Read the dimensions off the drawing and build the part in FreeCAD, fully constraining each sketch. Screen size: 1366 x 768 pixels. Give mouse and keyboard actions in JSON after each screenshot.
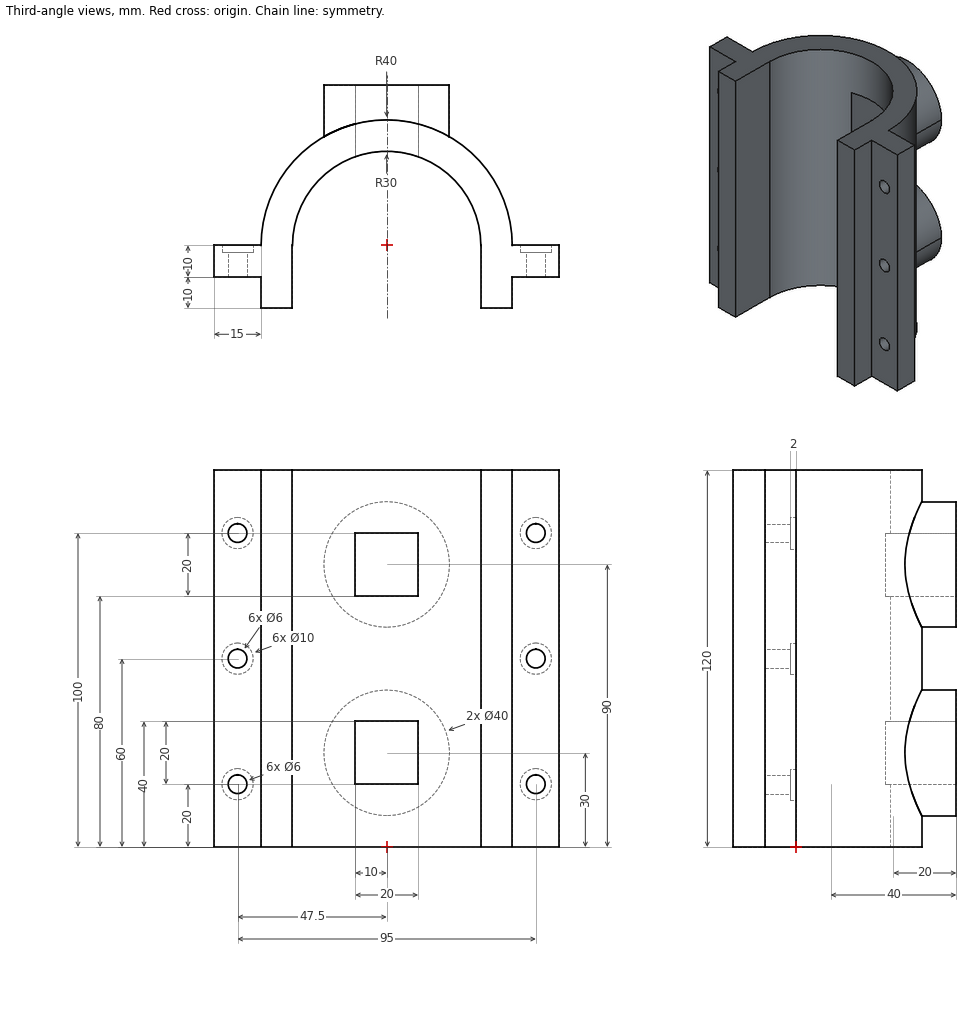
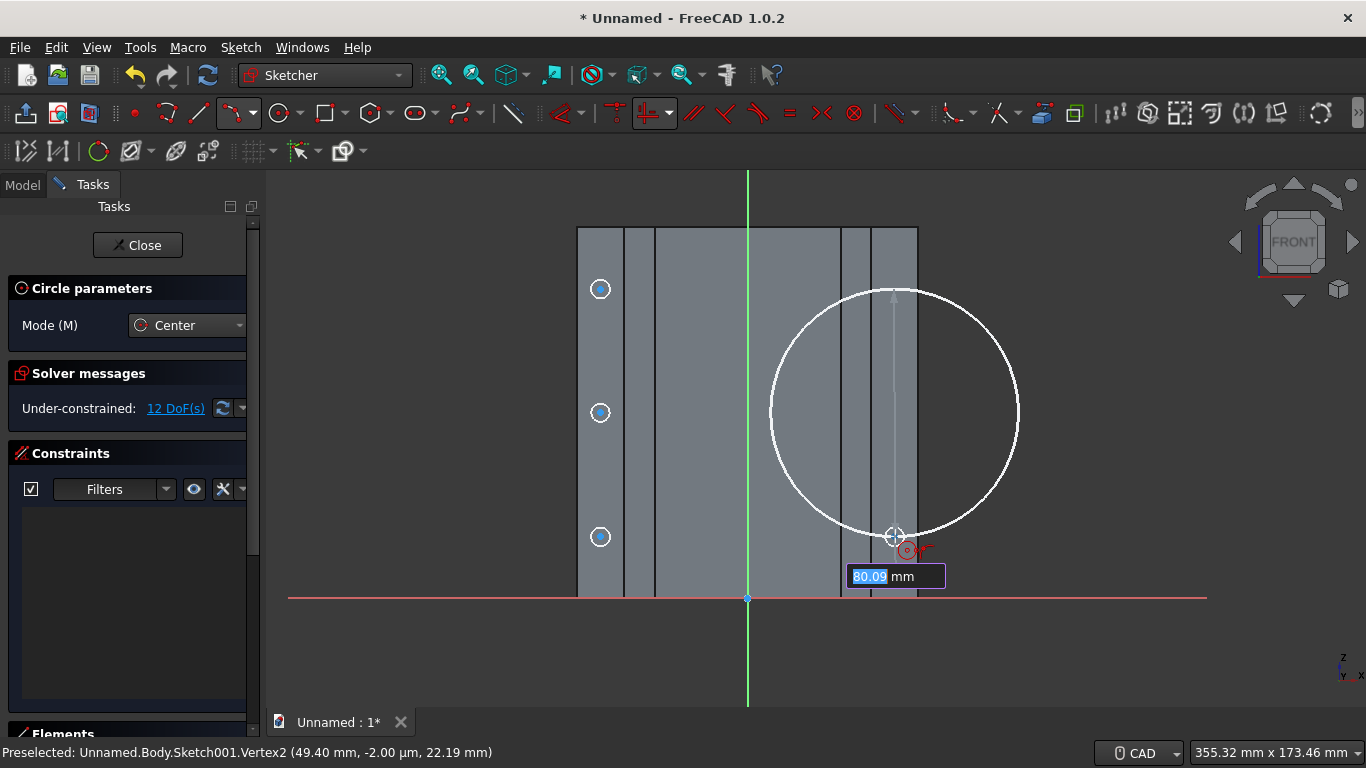
{"action": "scroll", "coordinate": [901, 406], "scroll_direction": "up", "scroll_amount": 3}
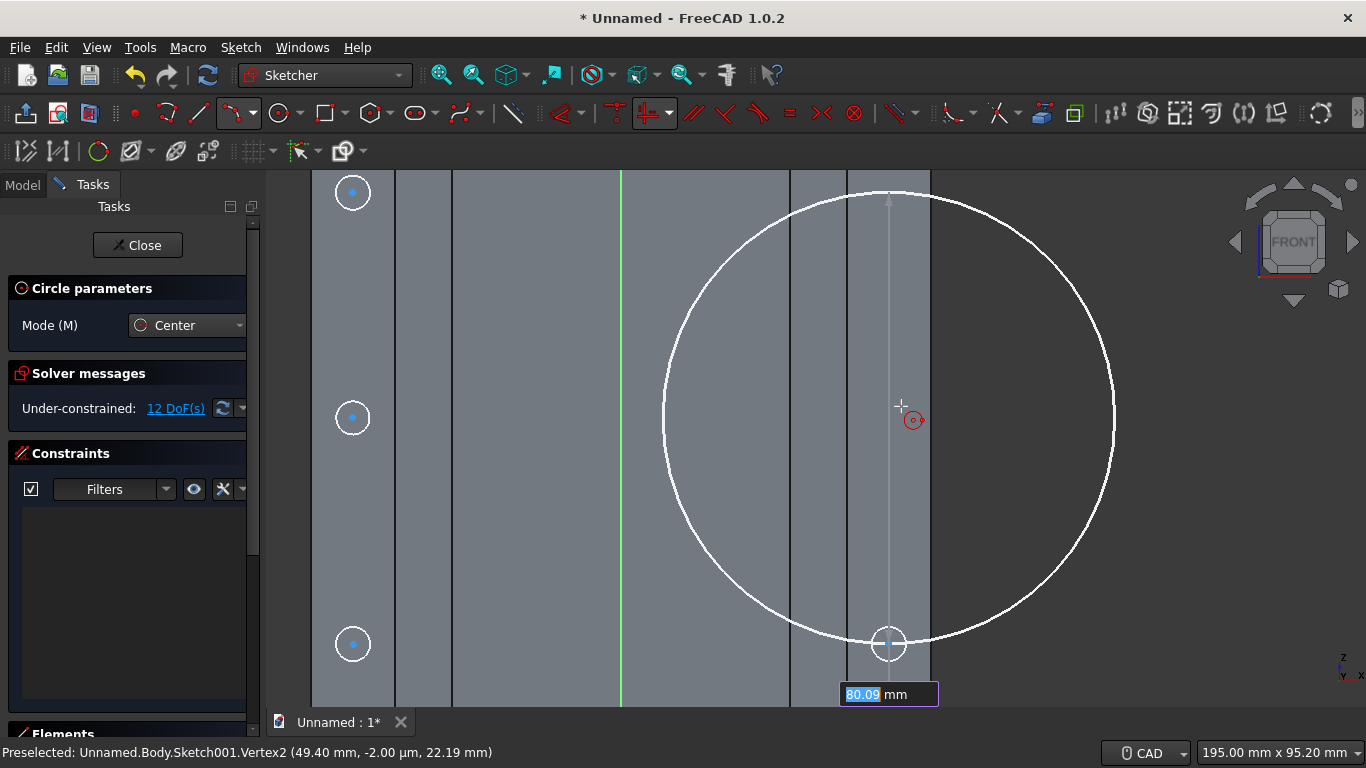
{"action": "left_click", "coordinate": [901, 406]}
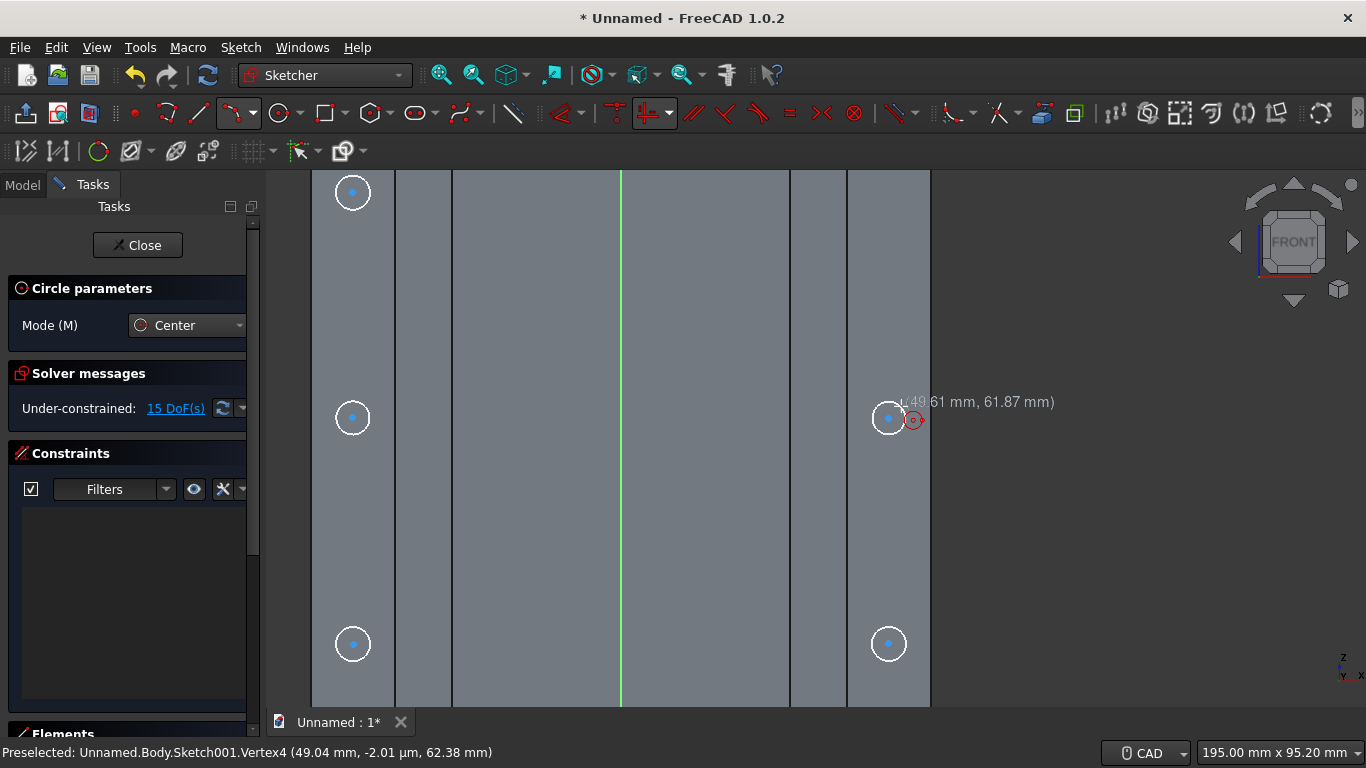
{"action": "scroll", "coordinate": [901, 406], "scroll_direction": "down", "scroll_amount": 3}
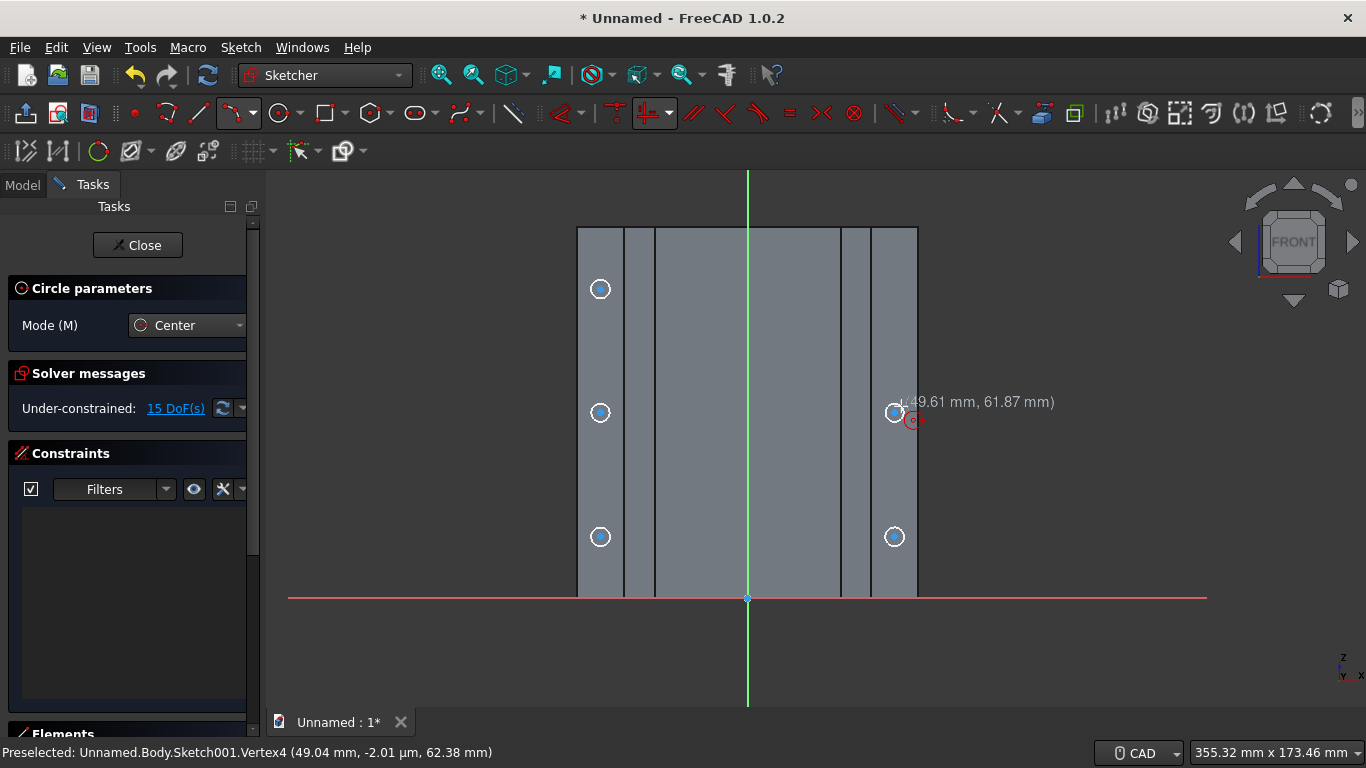
{"action": "scroll", "coordinate": [895, 289], "scroll_direction": "up", "scroll_amount": 5}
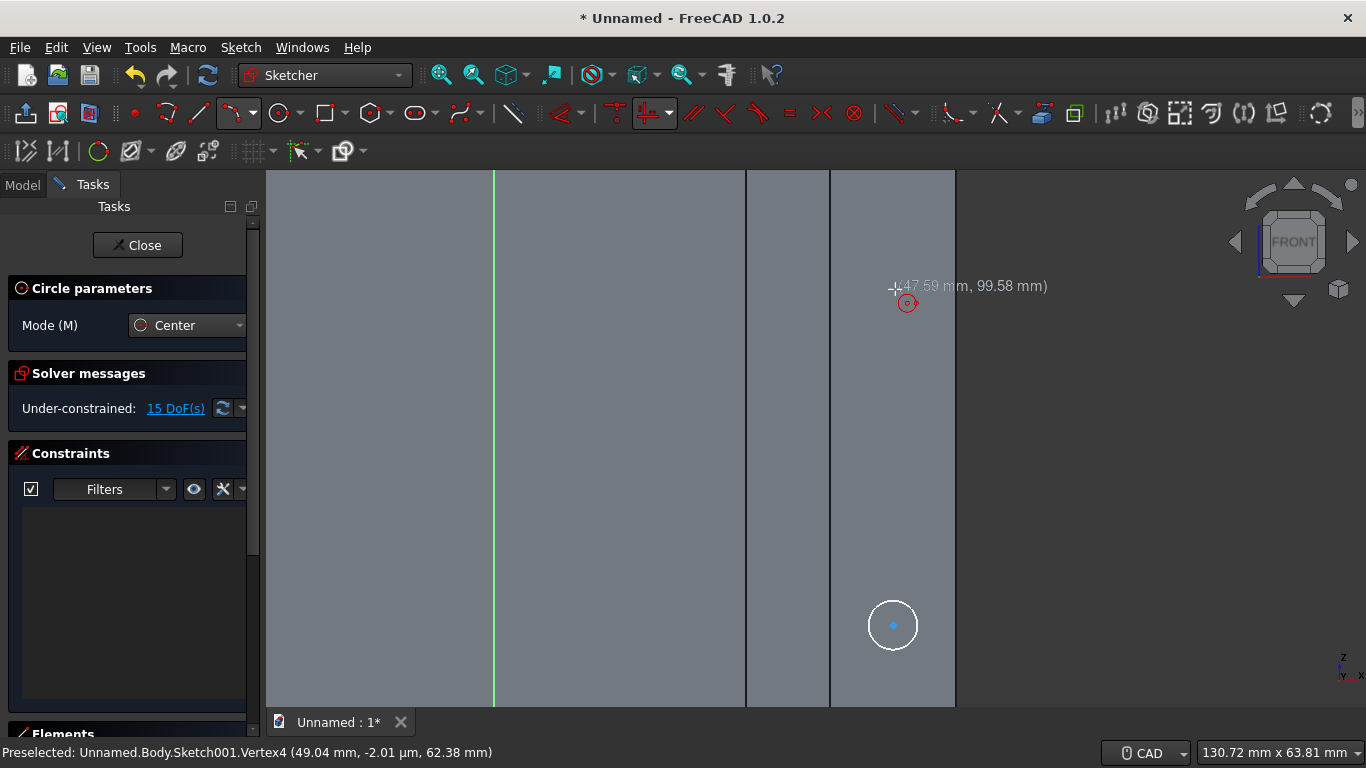
{"action": "left_click", "coordinate": [893, 288]}
{"action": "left_click", "coordinate": [911, 270]}
{"action": "key", "text": "Escape"}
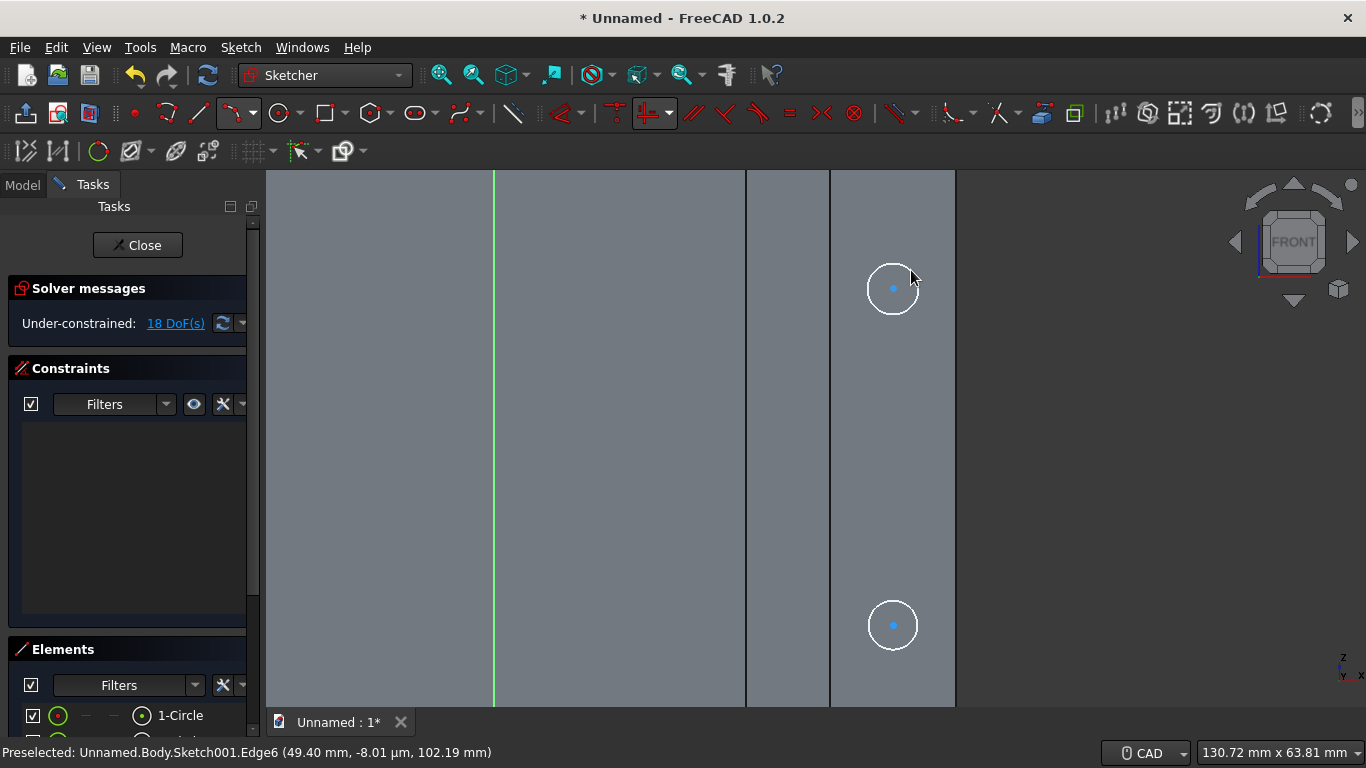
{"action": "scroll", "coordinate": [895, 289], "scroll_direction": "down", "scroll_amount": 5}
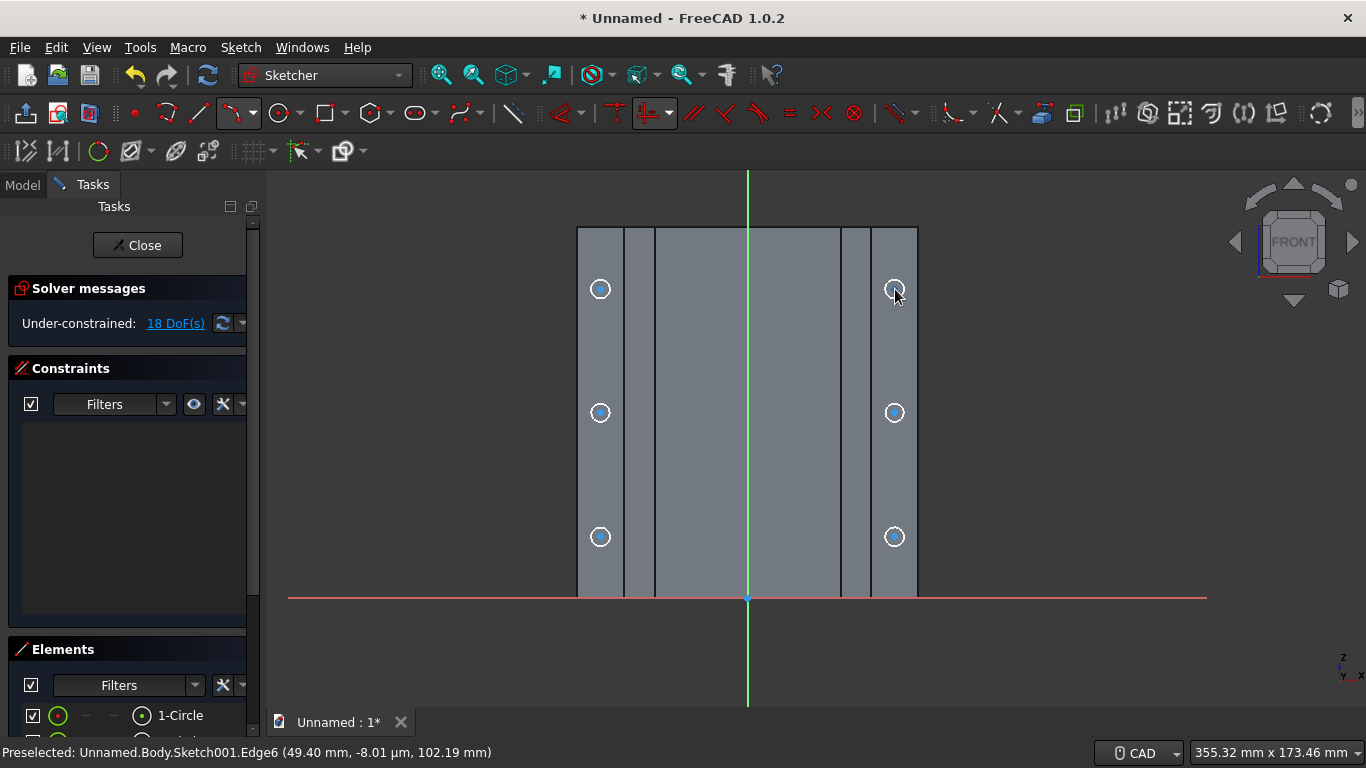
{"action": "scroll", "coordinate": [607, 530], "scroll_direction": "up", "scroll_amount": 2}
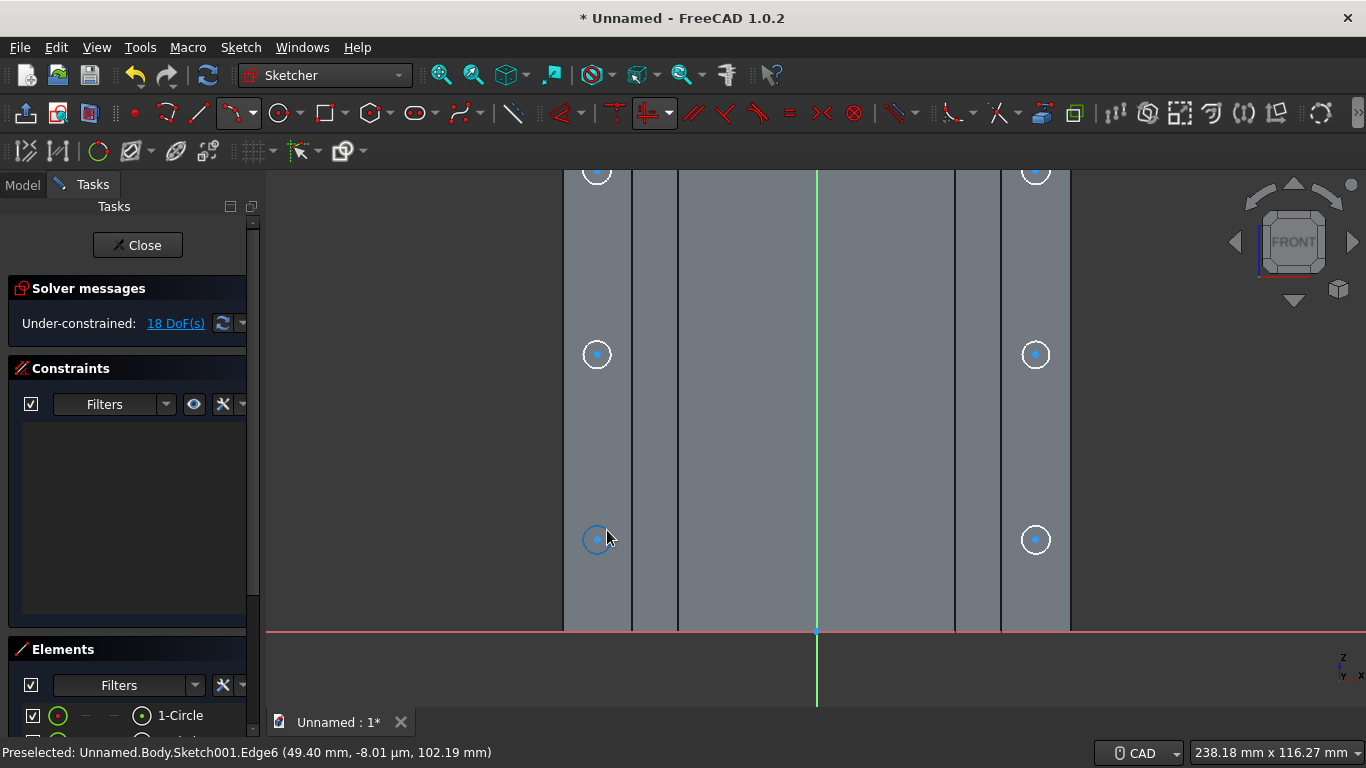
{"action": "left_click", "coordinate": [607, 530]}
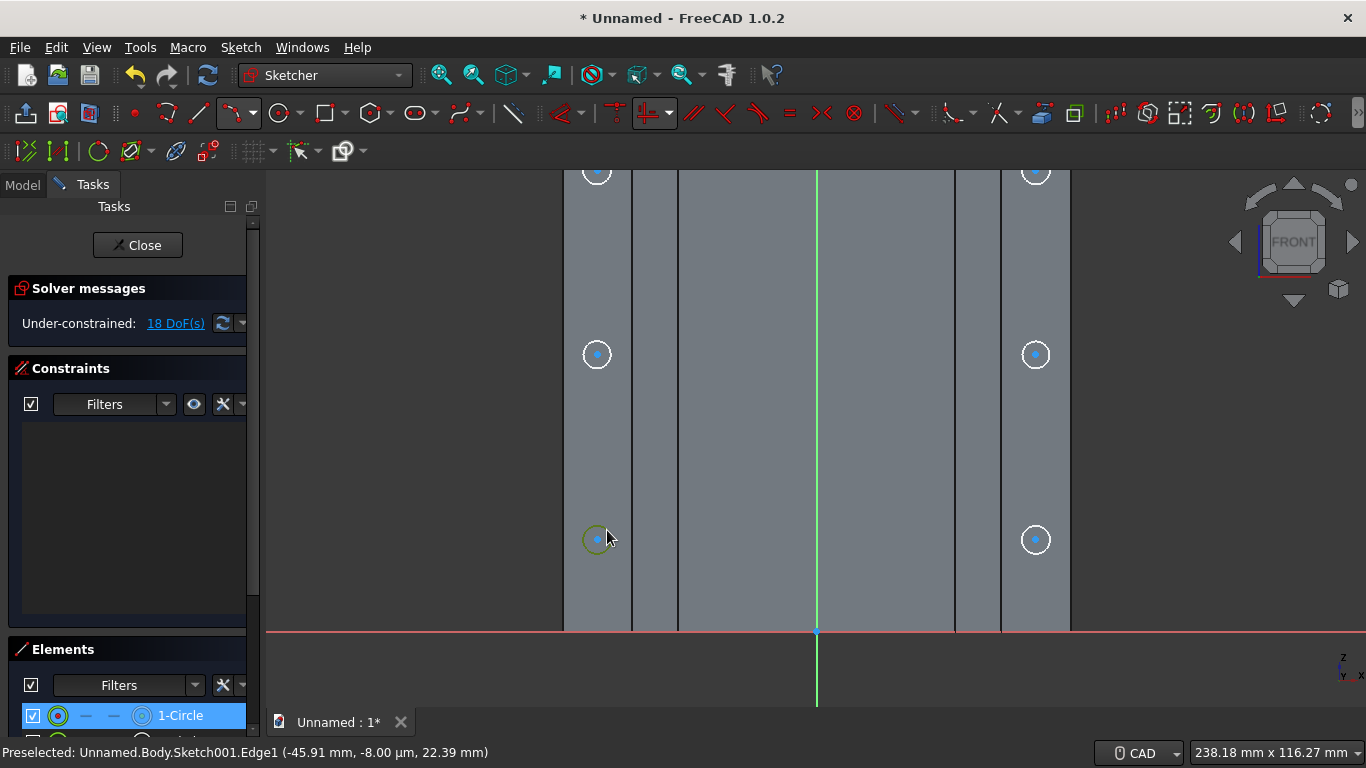
{"action": "scroll", "coordinate": [607, 530], "scroll_direction": "down", "scroll_amount": 2}